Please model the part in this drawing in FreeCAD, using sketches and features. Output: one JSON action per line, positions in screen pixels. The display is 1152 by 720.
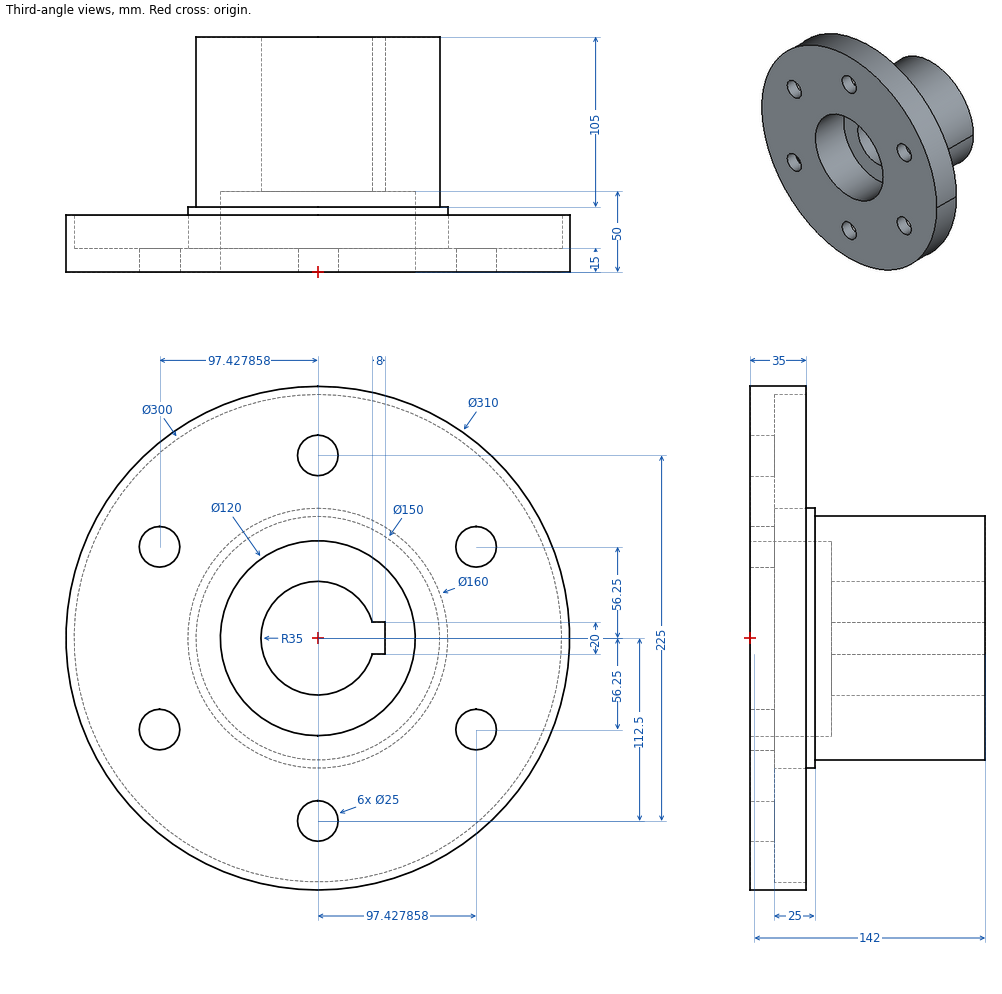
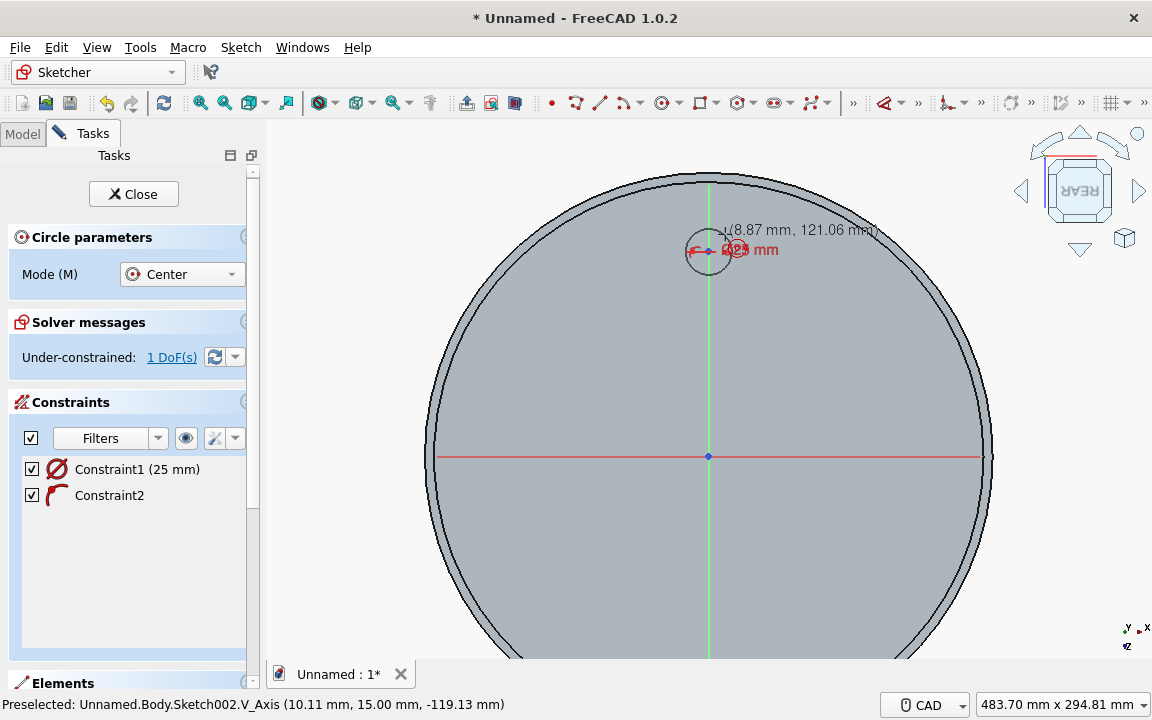
{"action": "left_click", "coordinate": [887, 354]}
{"action": "mouse_move", "coordinate": [903, 338]}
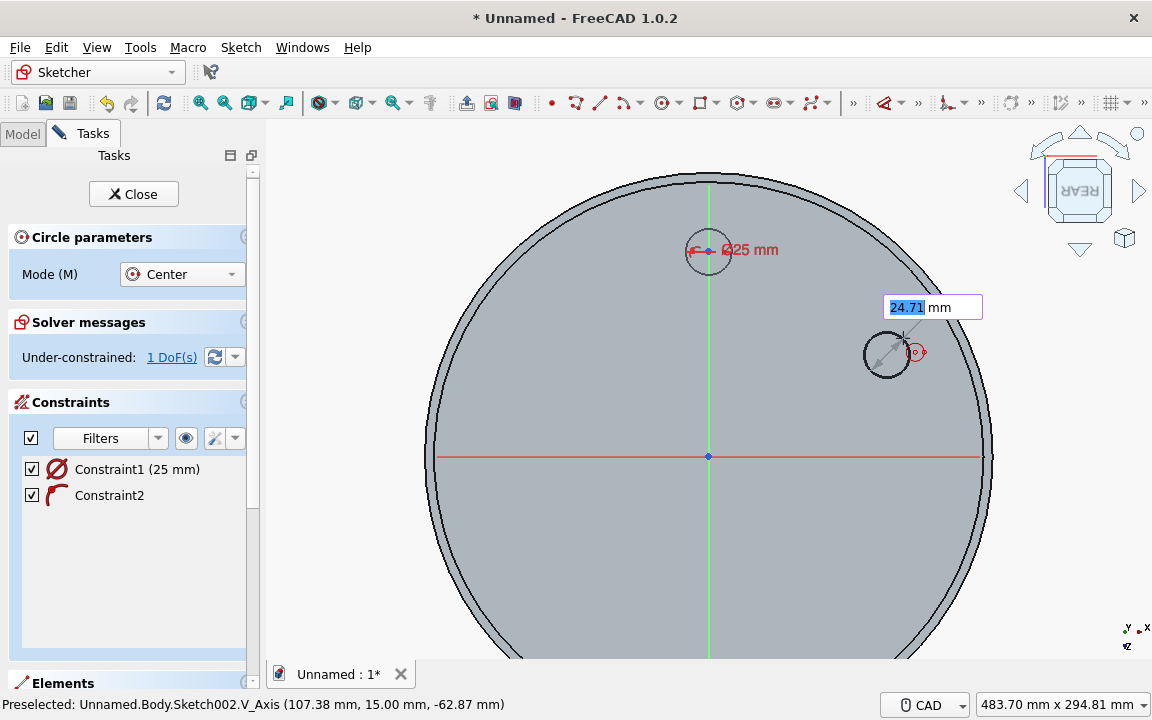
{"action": "type", "text": "25"}
{"action": "key", "text": "Return"}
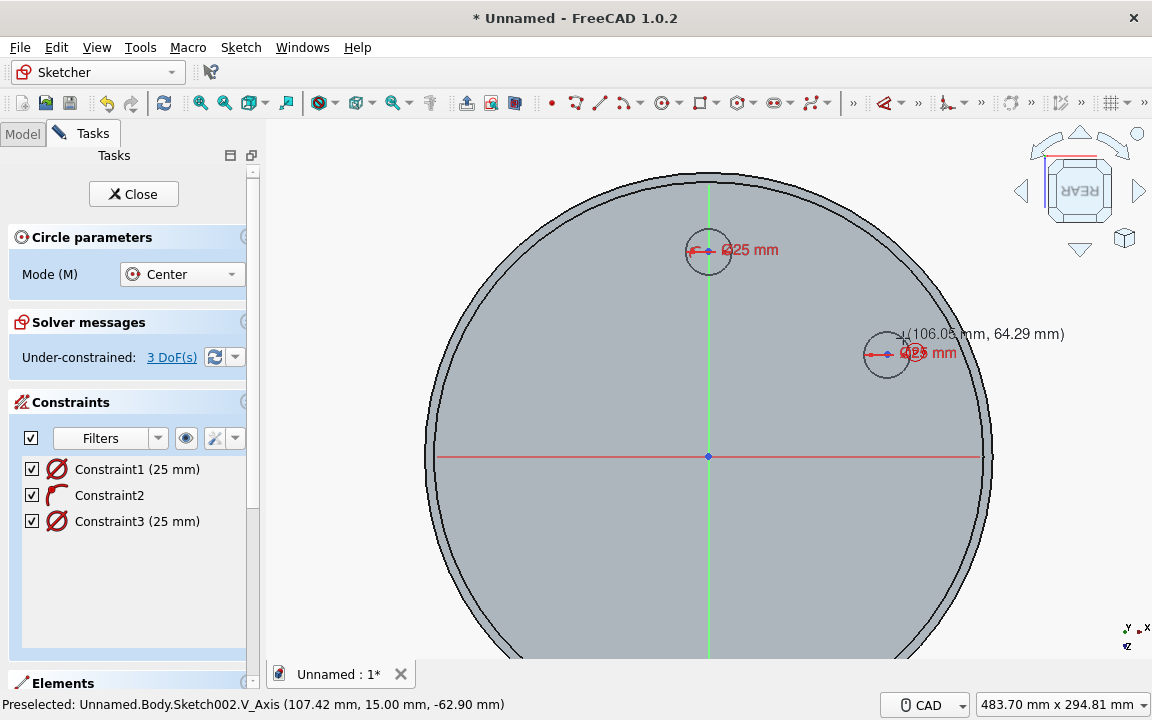
{"action": "left_click", "coordinate": [887, 560]}
{"action": "mouse_move", "coordinate": [903, 544]}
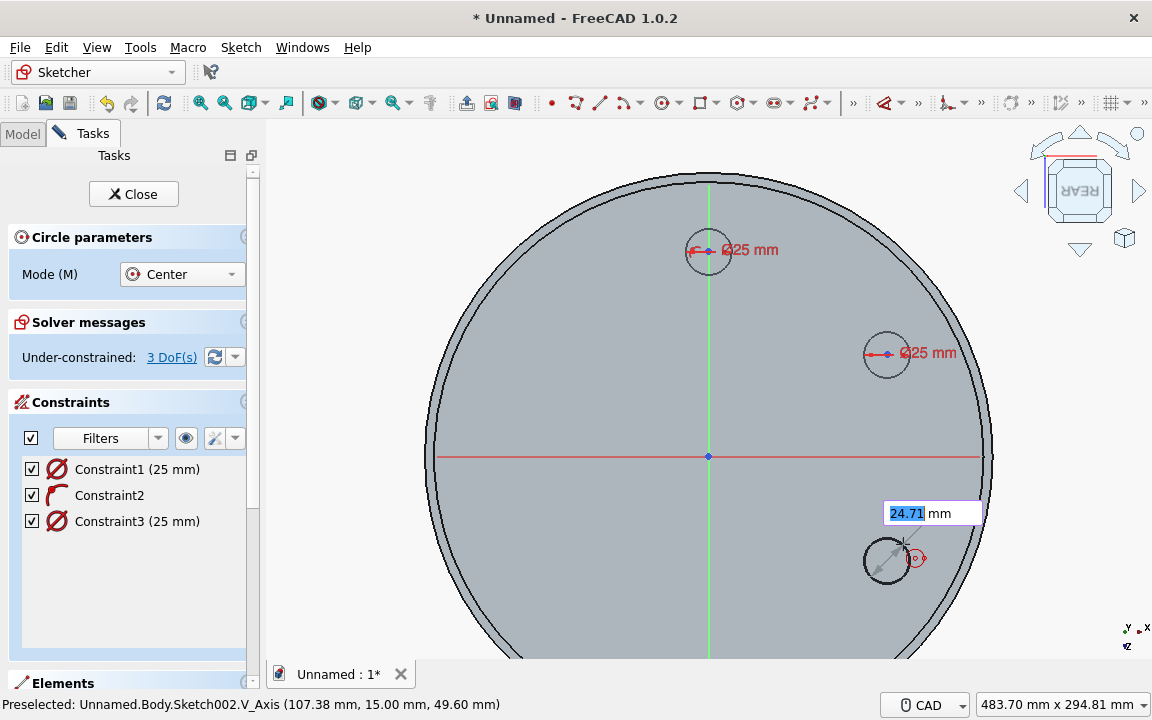
{"action": "type", "text": "25"}
{"action": "key", "text": "Return"}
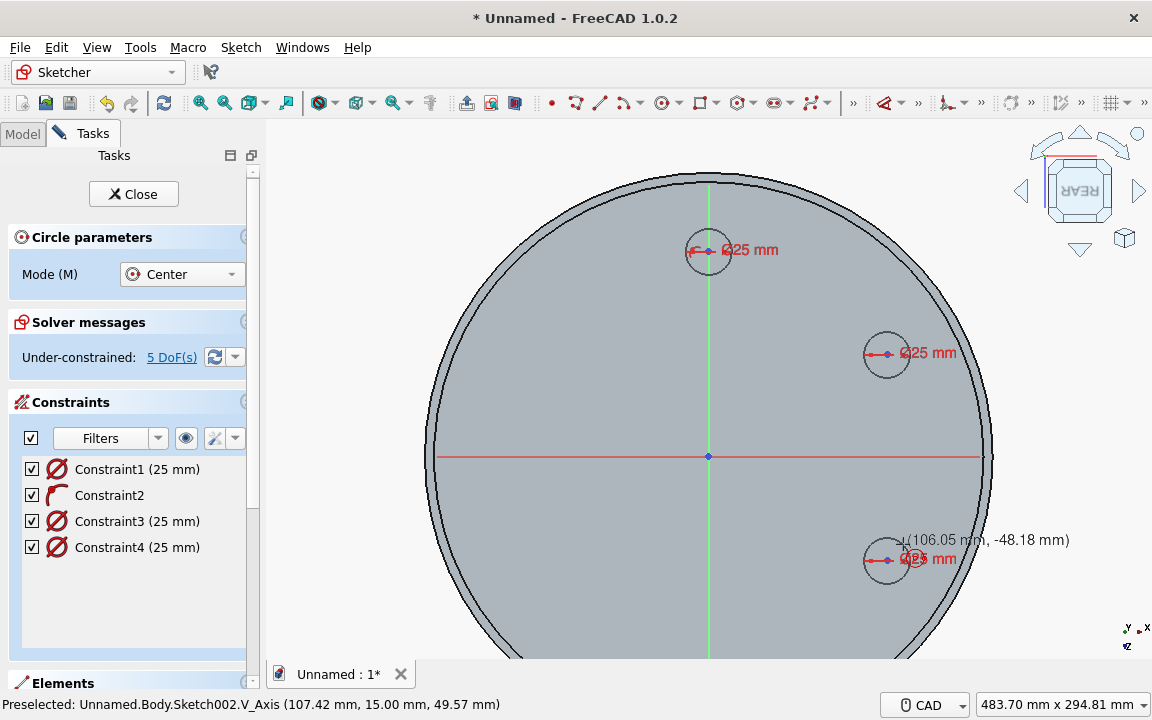
{"action": "scroll", "coordinate": [332, 147], "scroll_direction": "down", "scroll_amount": 1}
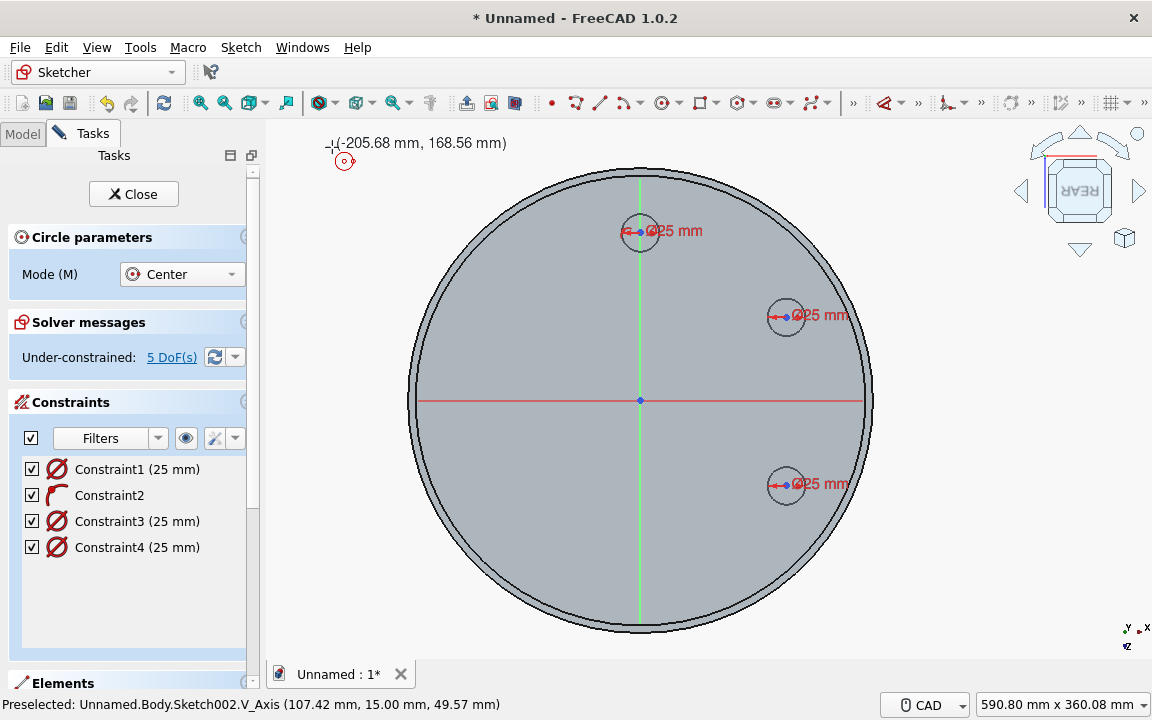
{"action": "left_click", "coordinate": [640, 569]}
{"action": "mouse_move", "coordinate": [658, 563]}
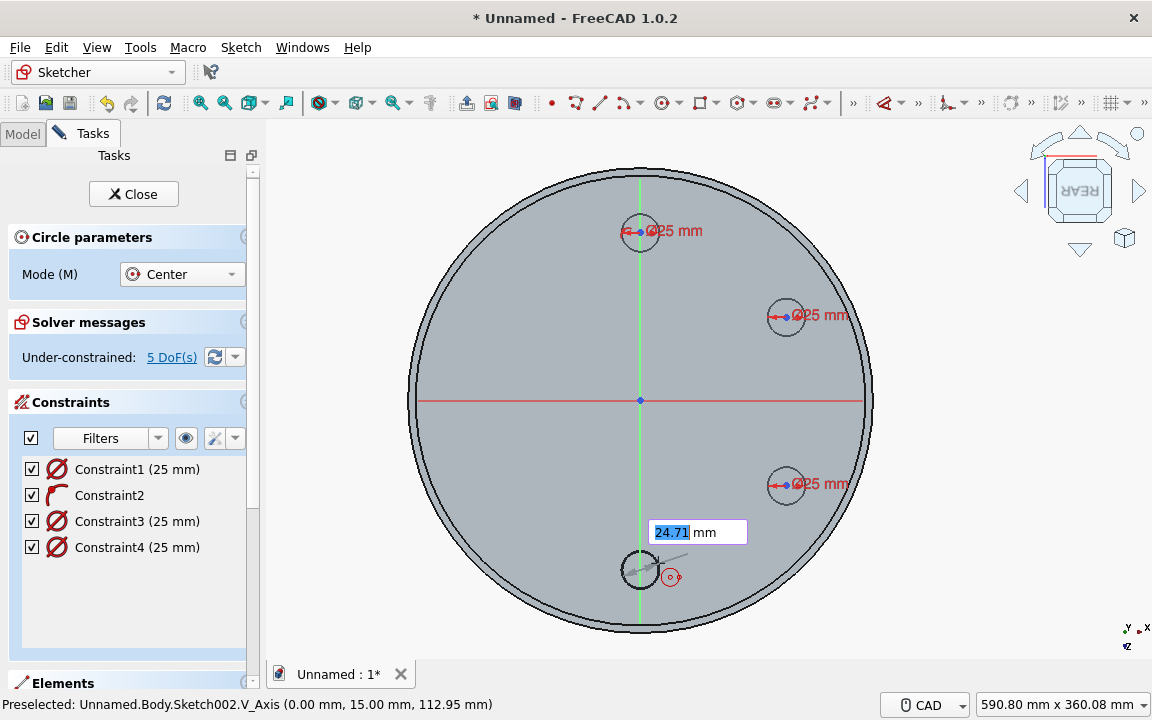
{"action": "type", "text": "25"}
{"action": "key", "text": "Return"}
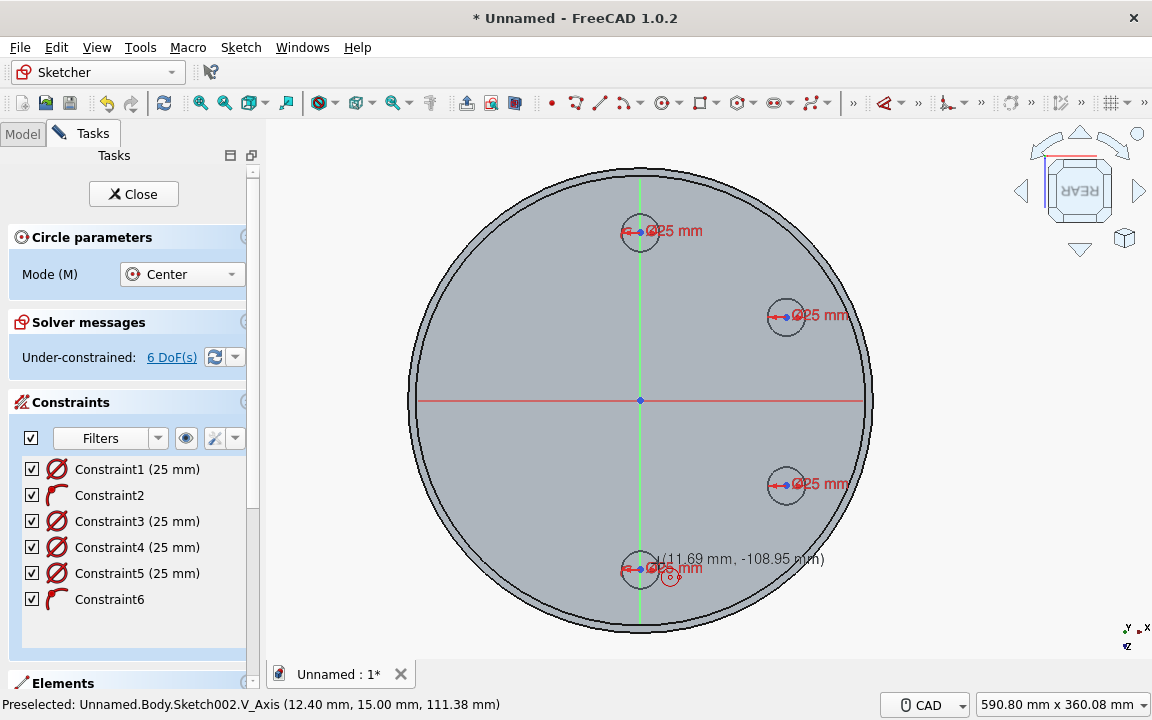
{"action": "left_click", "coordinate": [494, 485]}
{"action": "mouse_move", "coordinate": [508, 472]}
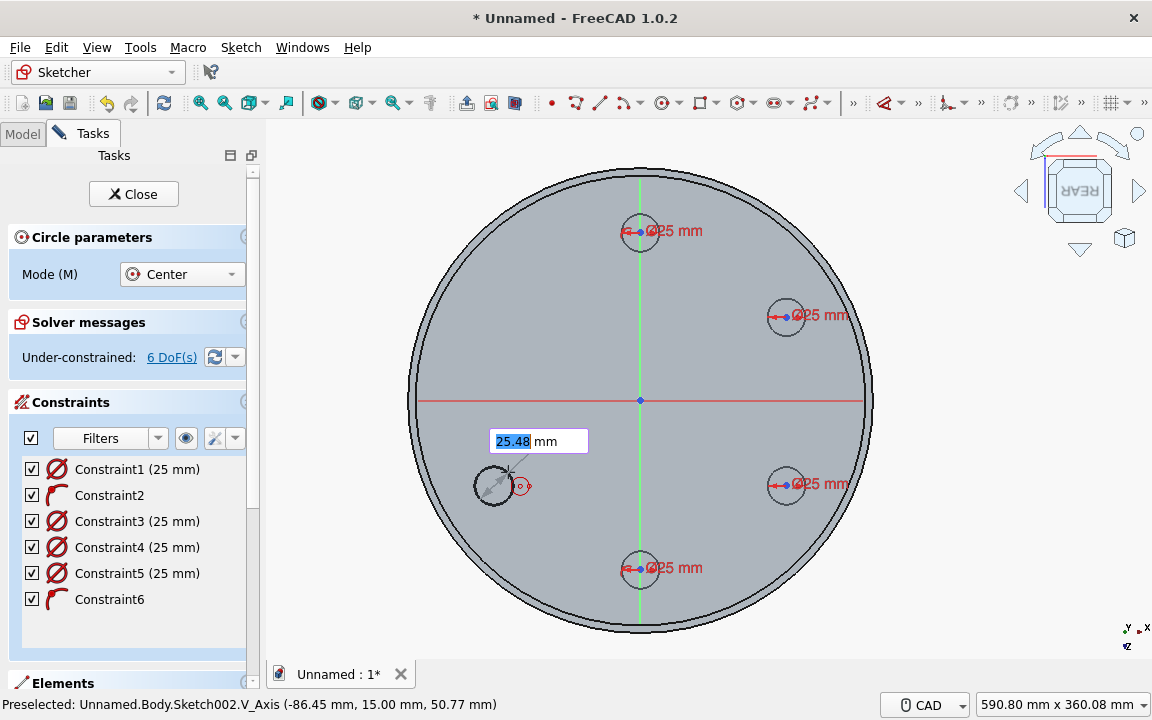
{"action": "type", "text": "25"}
{"action": "key", "text": "Return"}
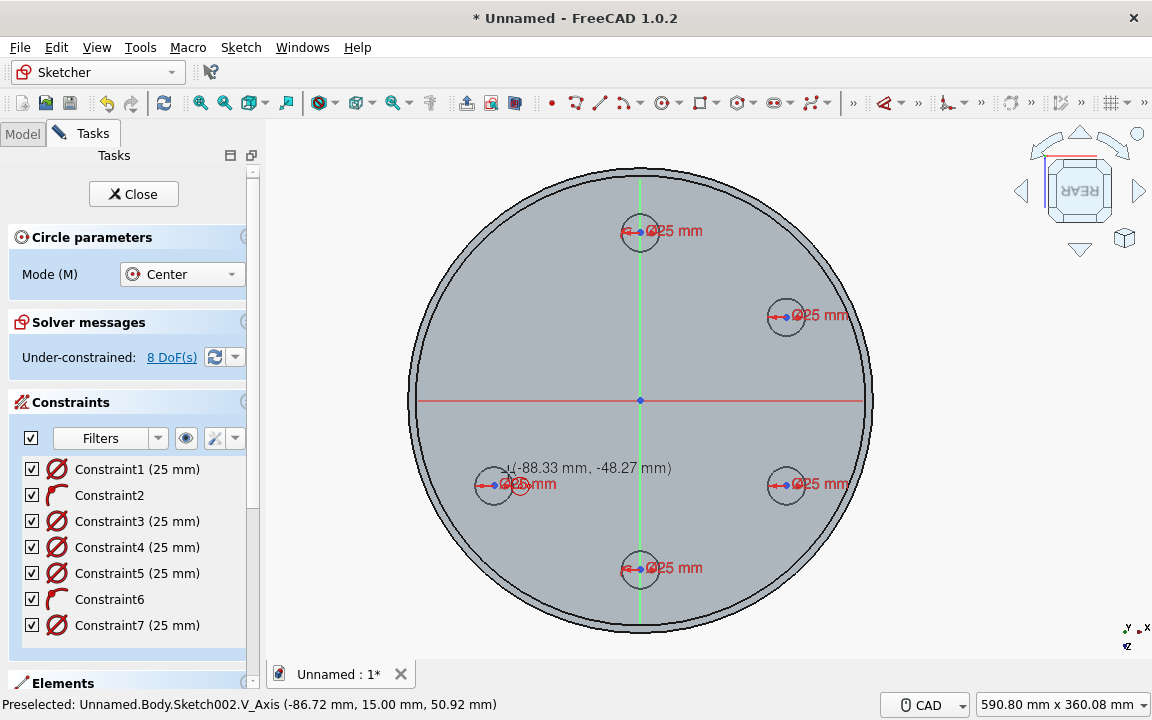
{"action": "left_click", "coordinate": [494, 316]}
{"action": "mouse_move", "coordinate": [508, 303]}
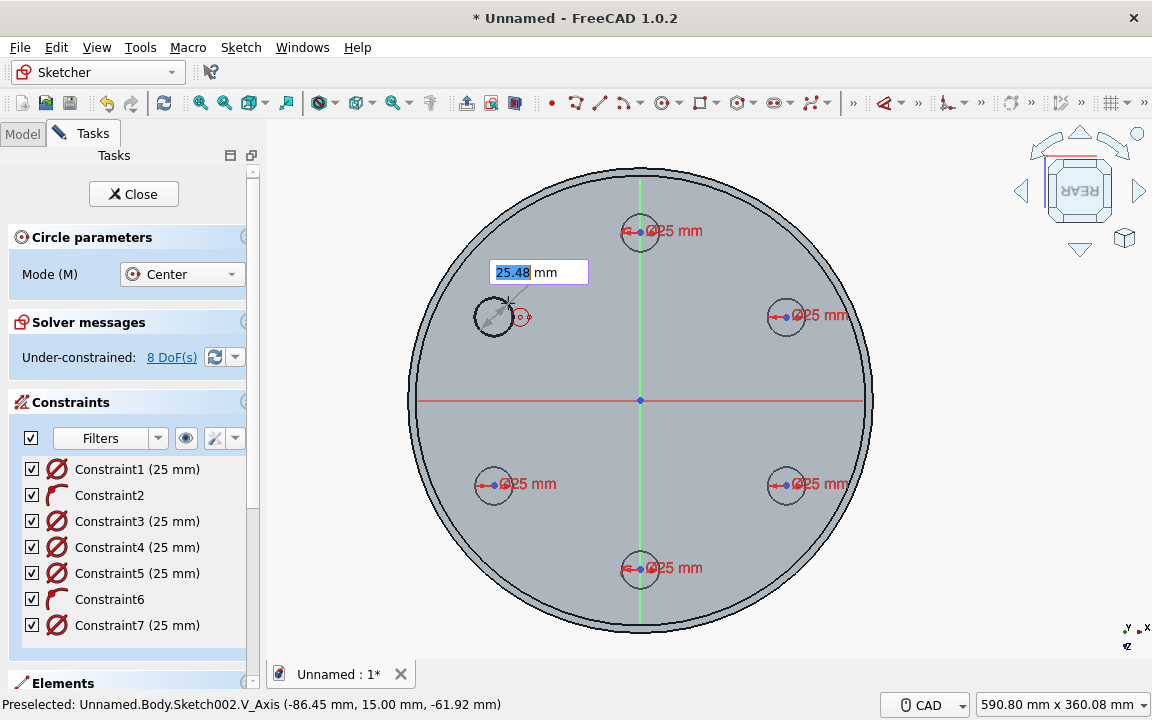
{"action": "type", "text": "25"}
{"action": "key", "text": "Return"}
{"action": "key", "text": "Escape"}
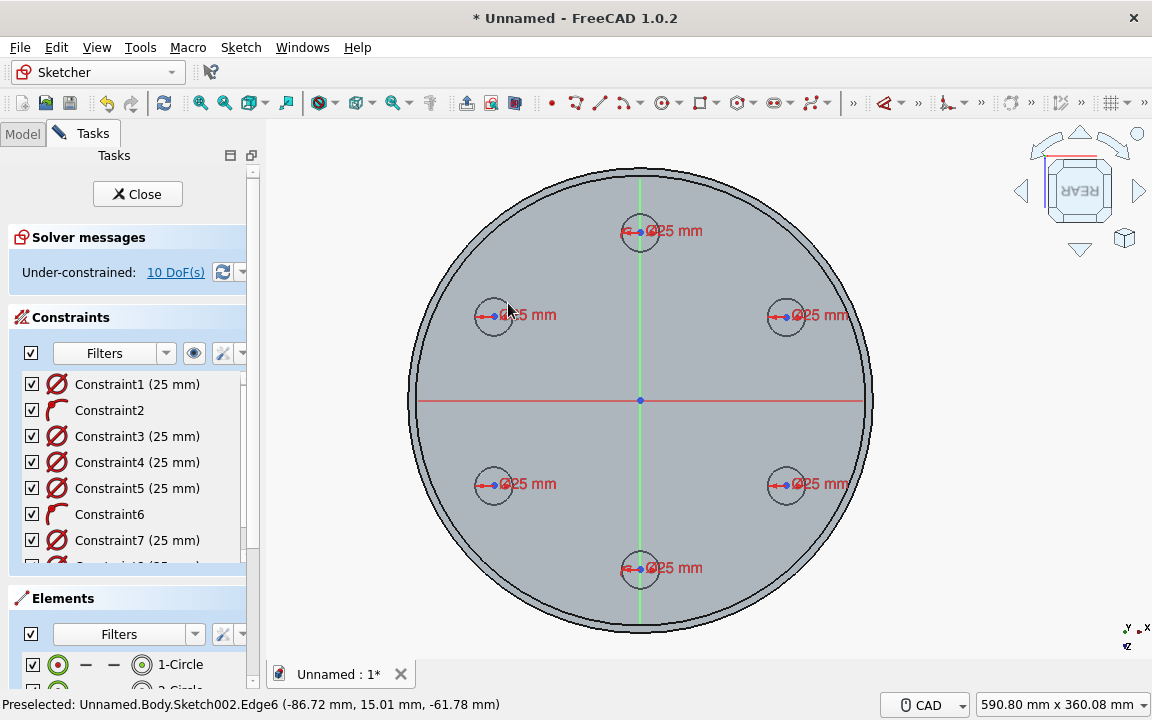
{"action": "left_click", "coordinate": [786, 317]}